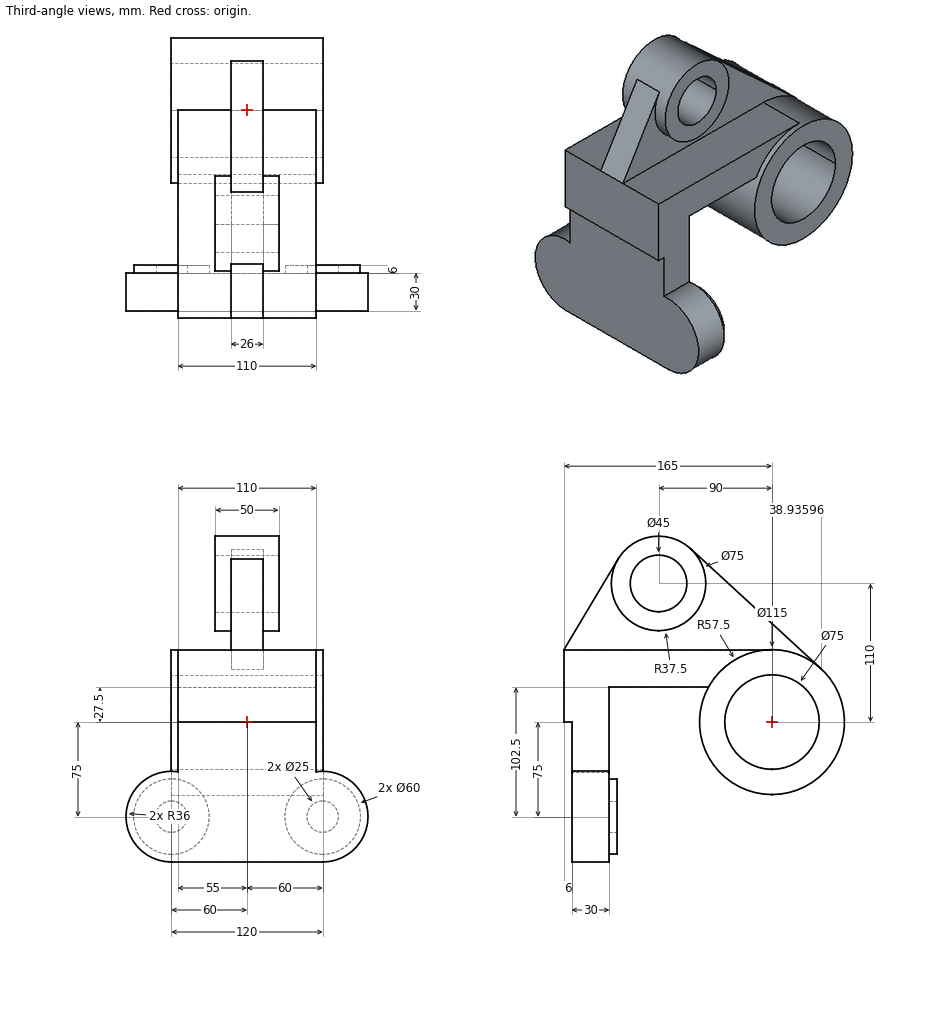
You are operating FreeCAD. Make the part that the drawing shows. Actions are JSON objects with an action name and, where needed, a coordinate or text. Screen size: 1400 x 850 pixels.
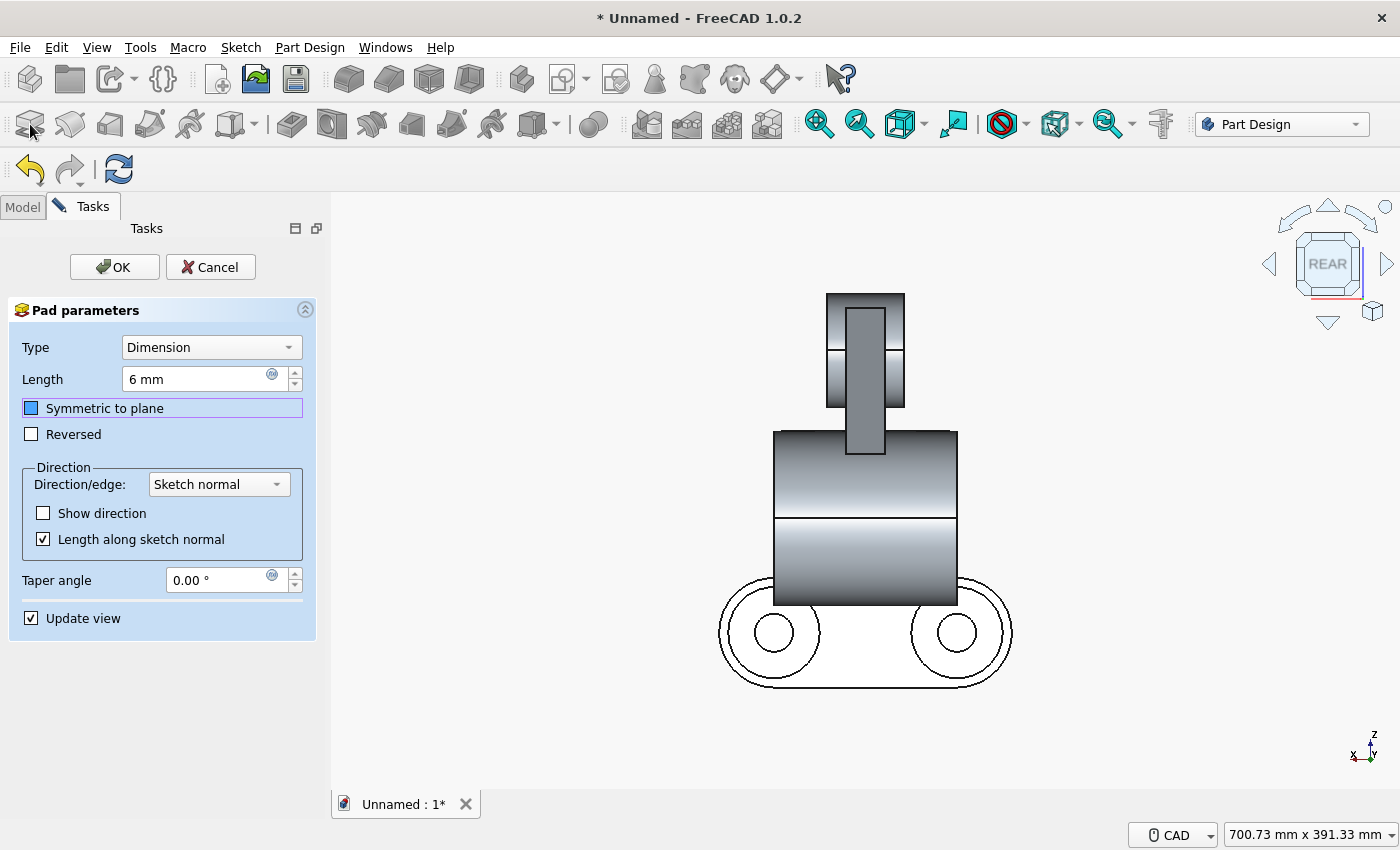
{"action": "left_click", "coordinate": [115, 267]}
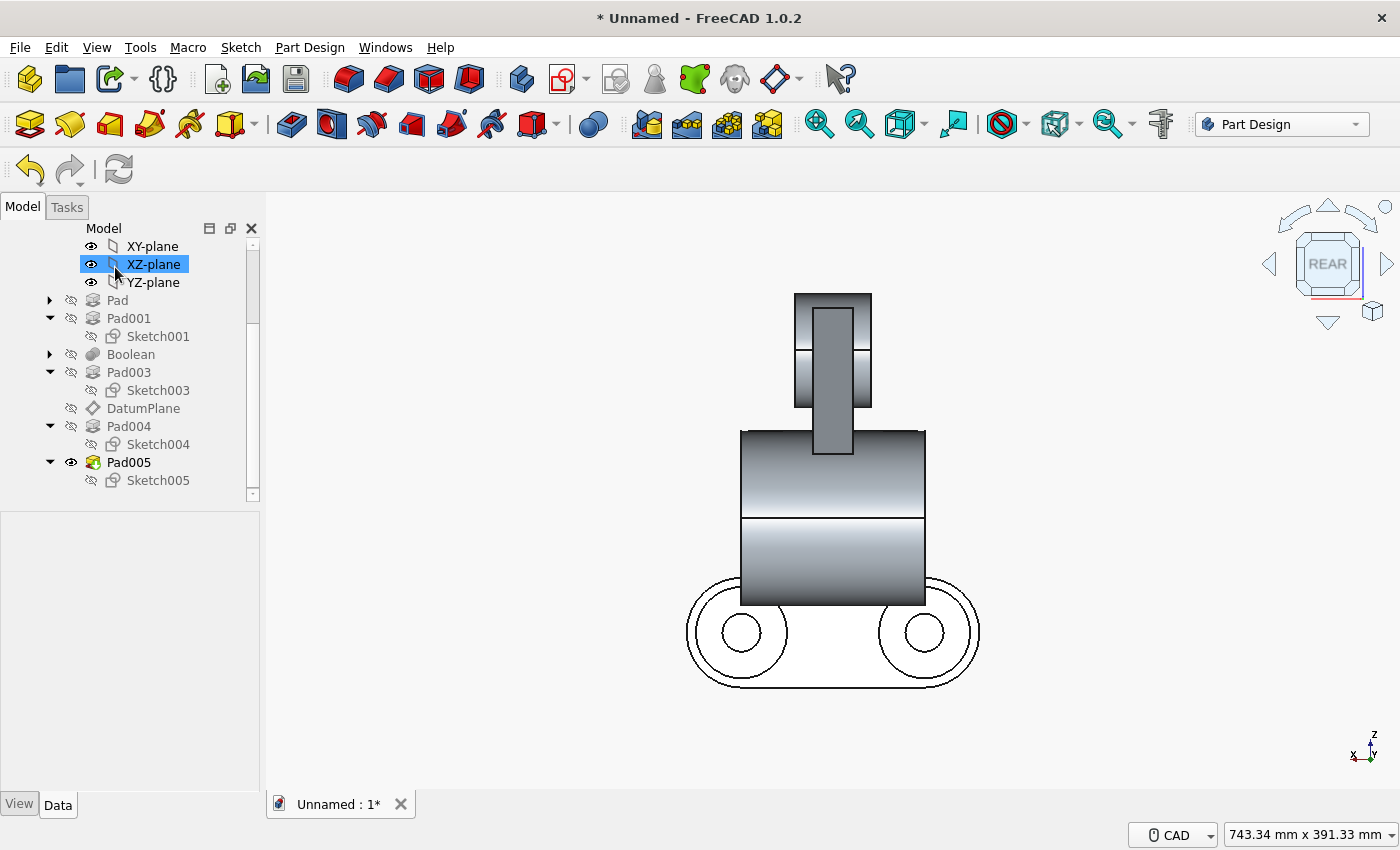
{"action": "key", "text": "0"}